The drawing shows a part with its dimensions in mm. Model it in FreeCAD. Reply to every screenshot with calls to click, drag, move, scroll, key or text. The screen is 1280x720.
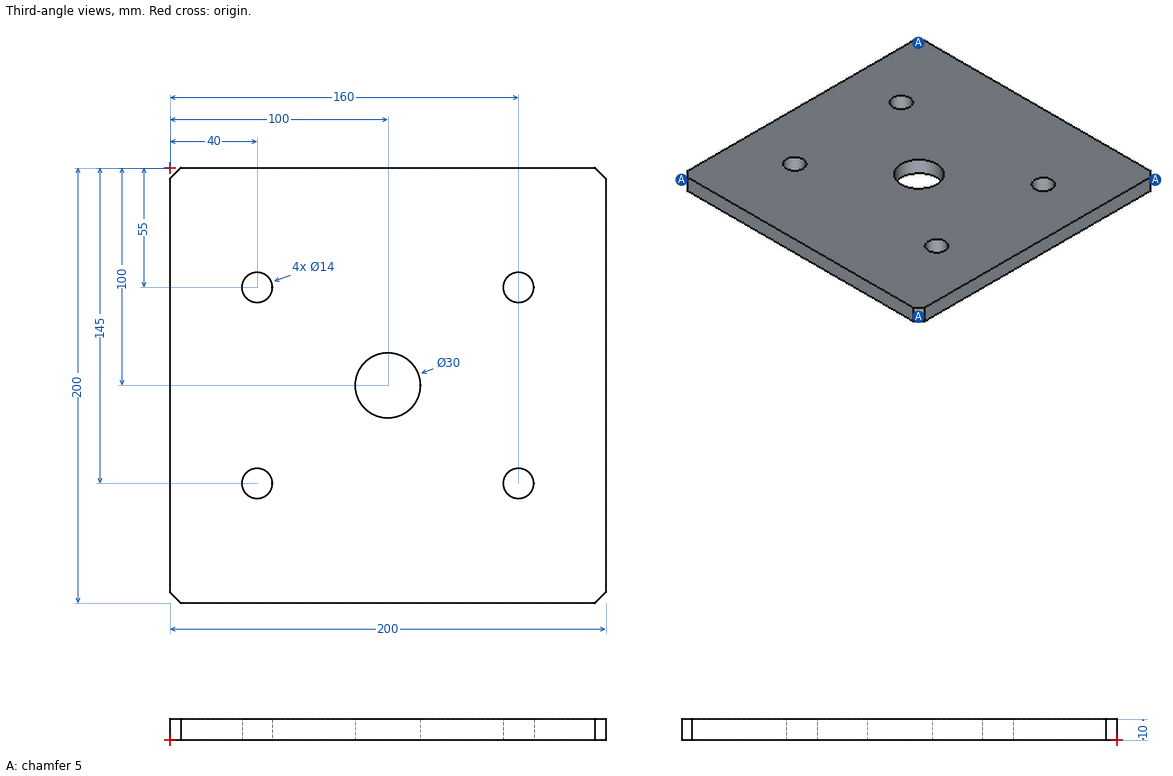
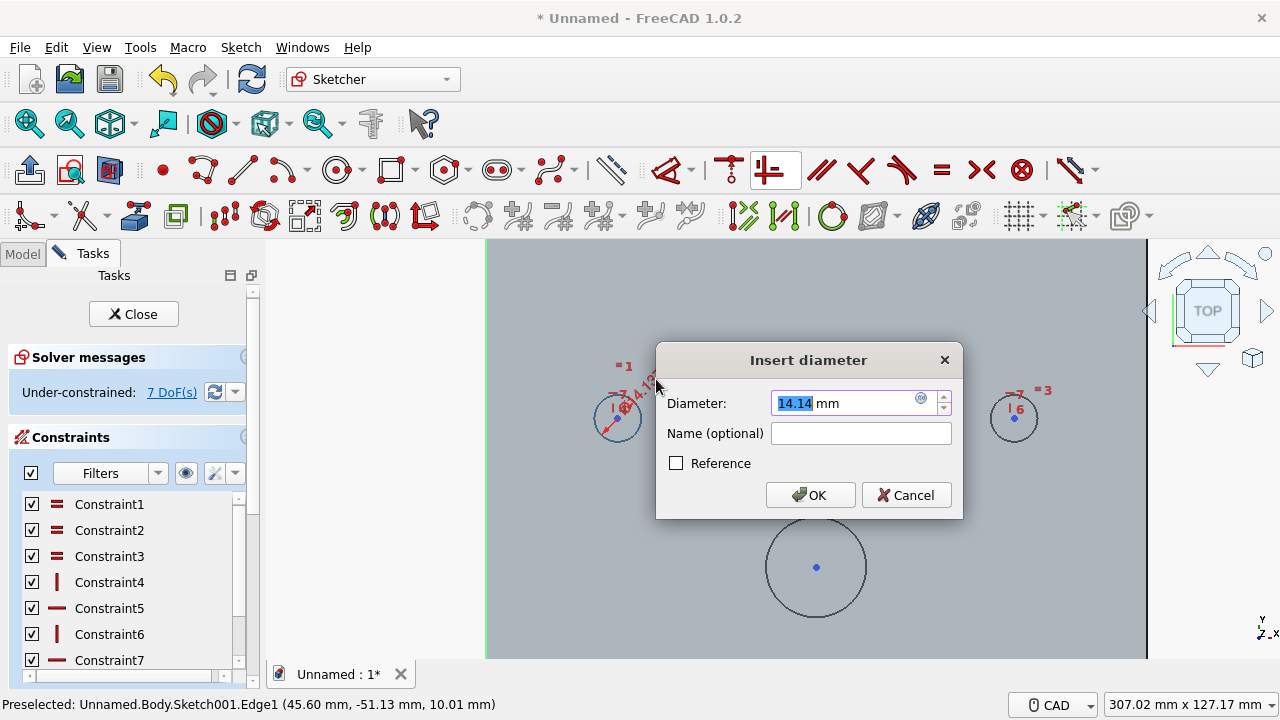
text(14)
key(Return)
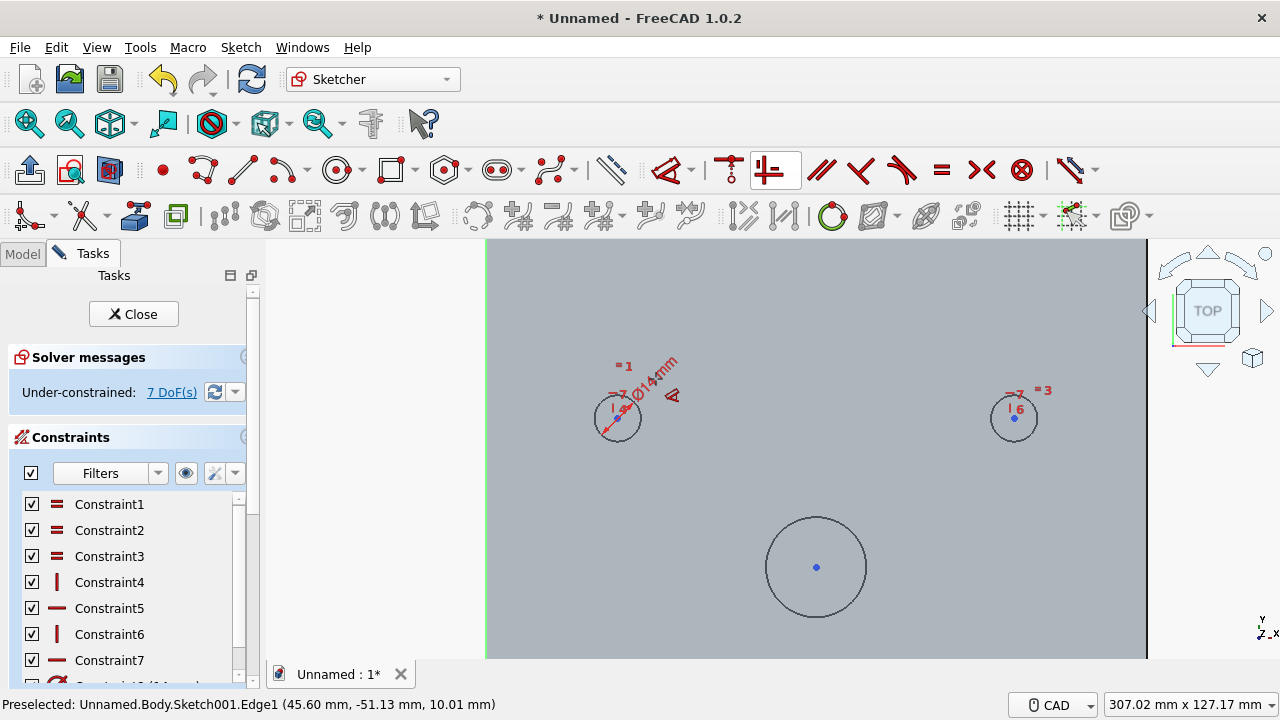
click(851, 532)
click(874, 509)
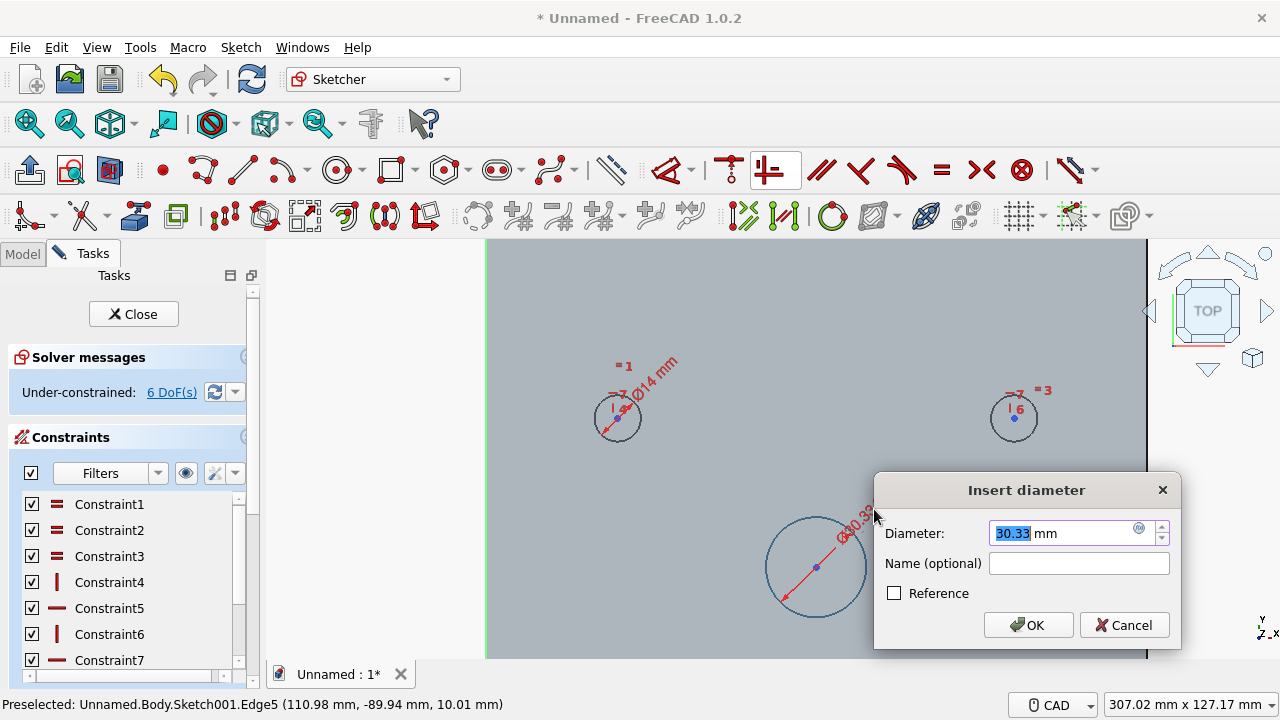
text(30)
key(Return)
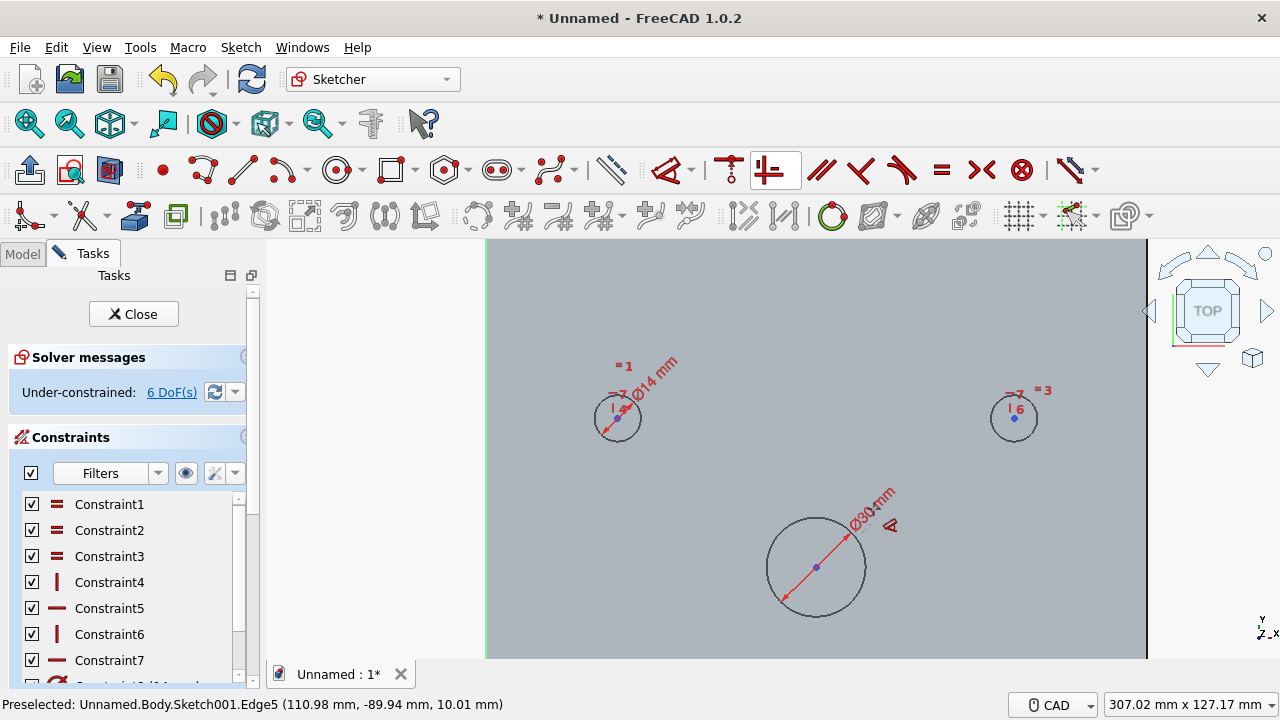
click(618, 418)
click(552, 452)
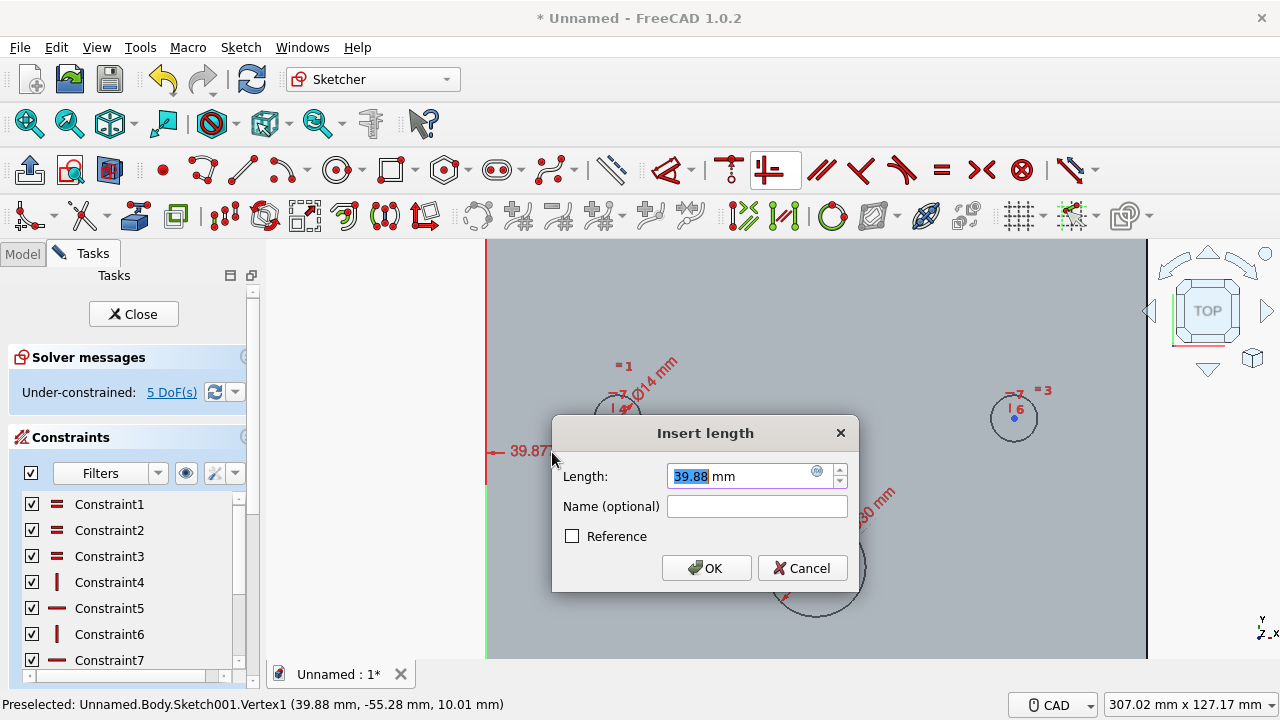
text(40)
key(Return)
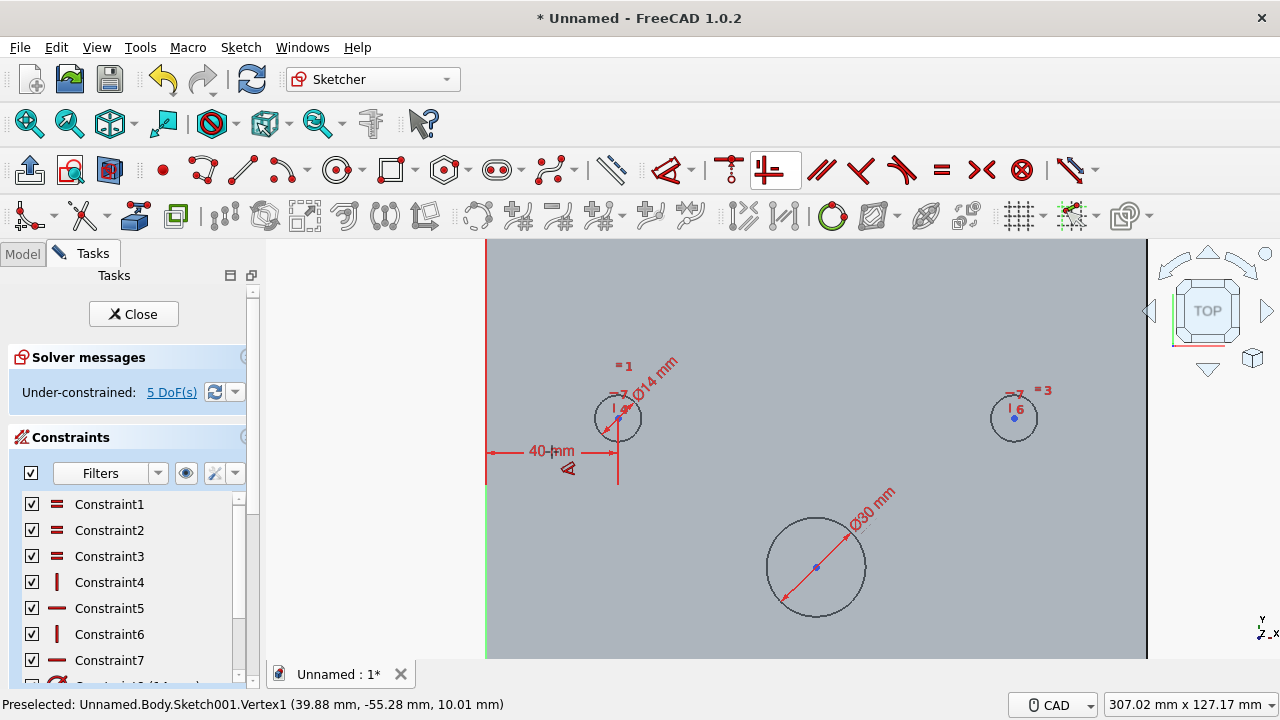
click(618, 418)
click(452, 343)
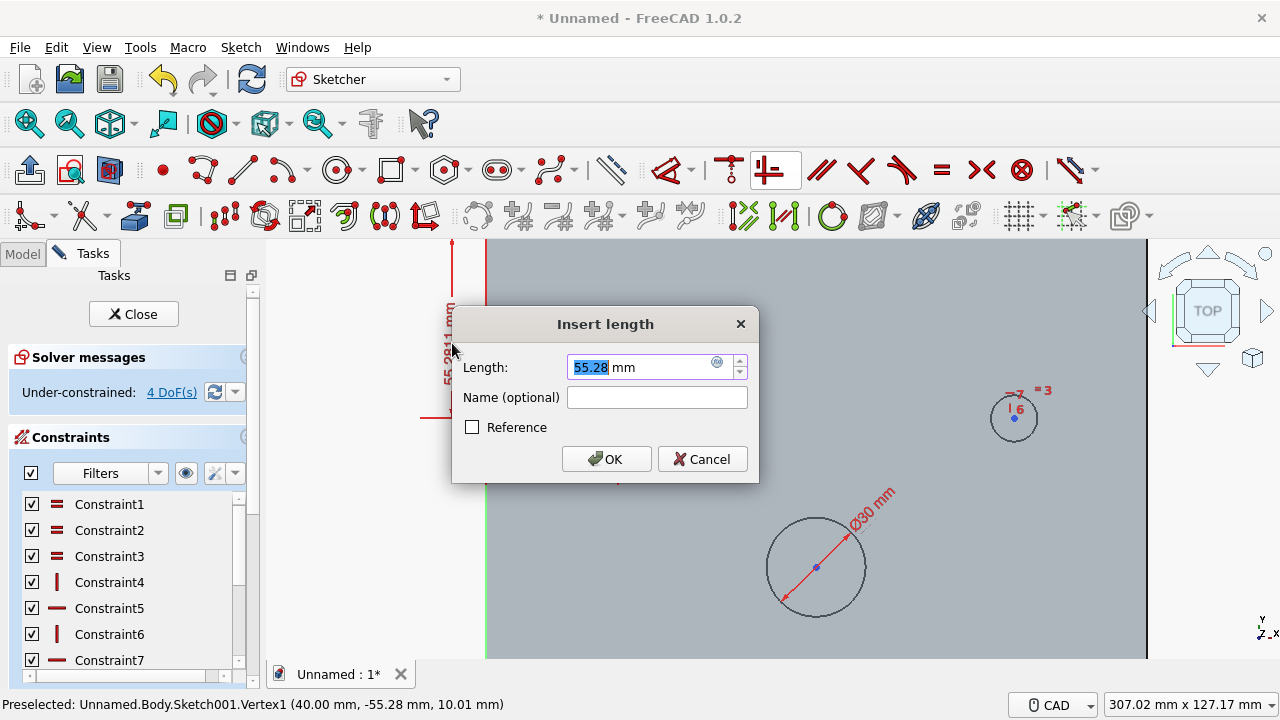
text(55)
key(Return)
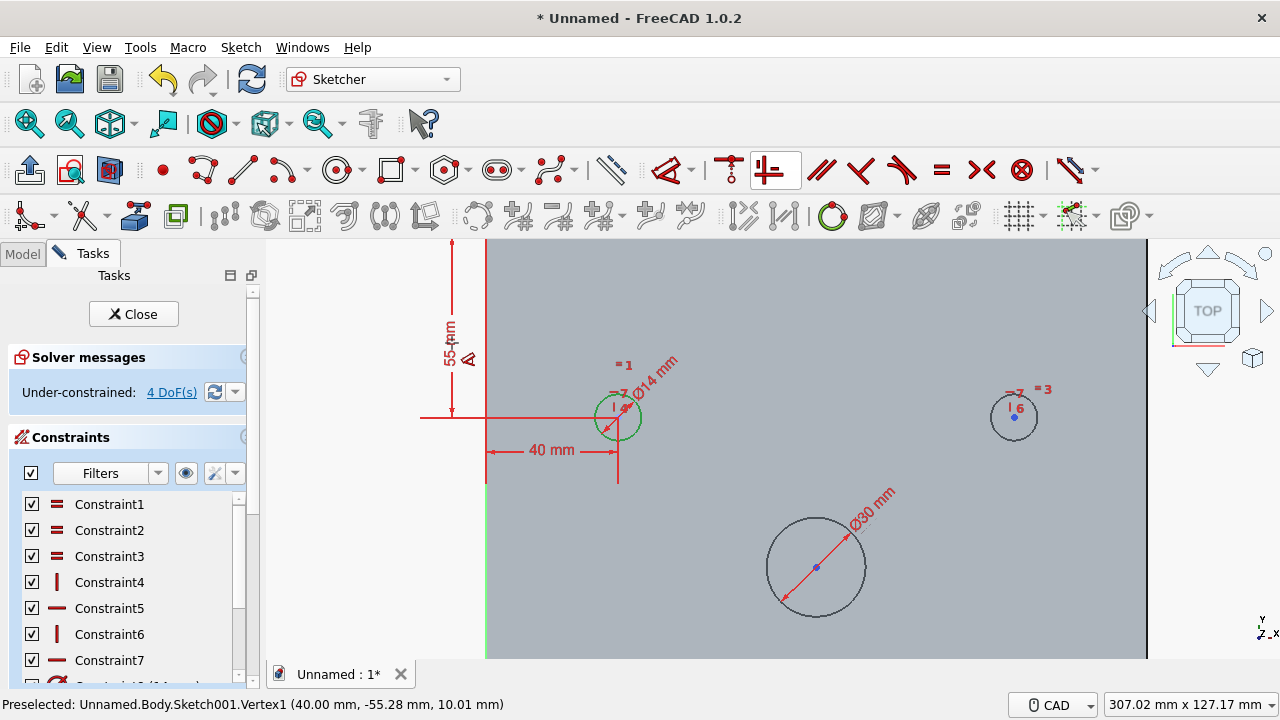
scroll(635, 403, down, 3)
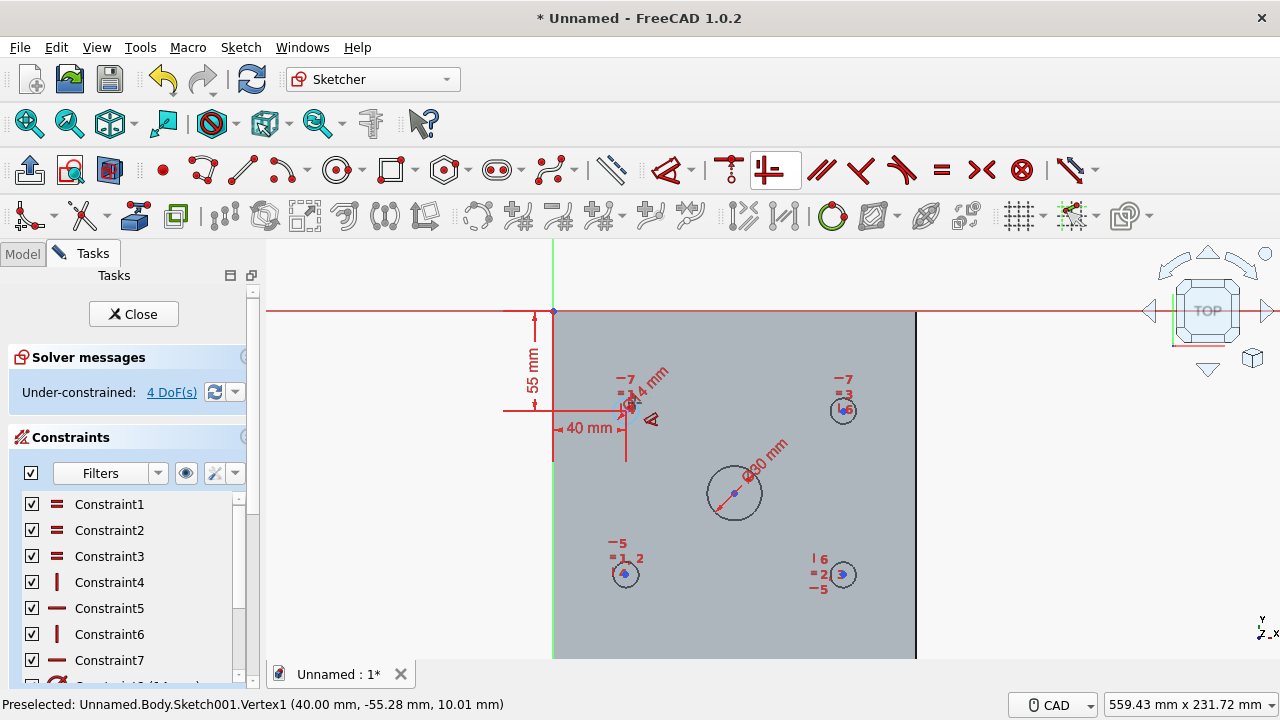
click(626, 575)
click(519, 443)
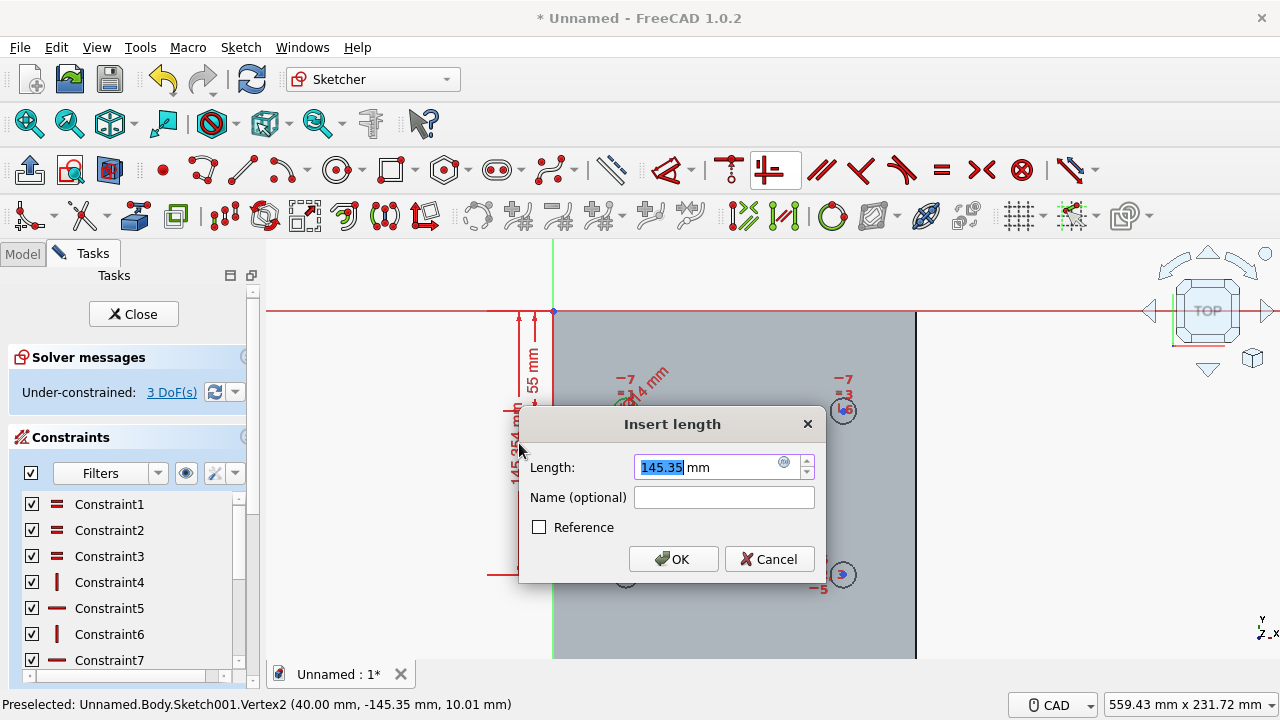
text(145)
key(Return)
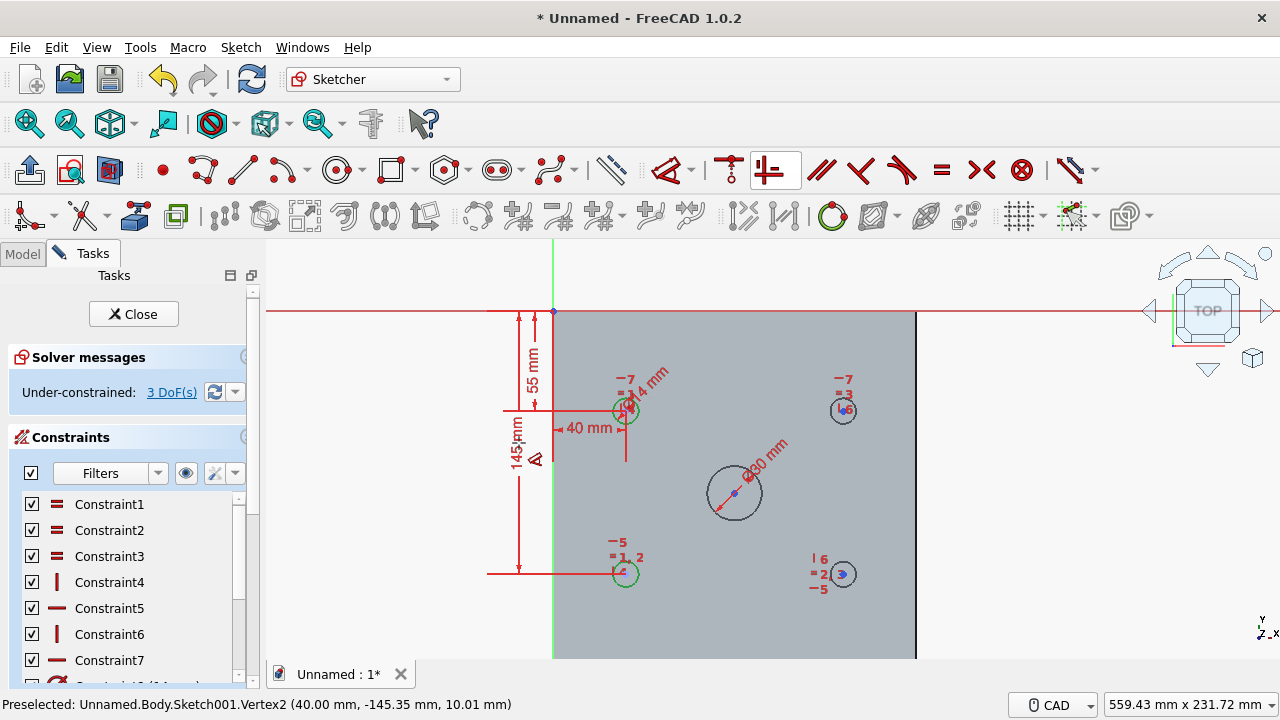
click(843, 574)
click(698, 277)